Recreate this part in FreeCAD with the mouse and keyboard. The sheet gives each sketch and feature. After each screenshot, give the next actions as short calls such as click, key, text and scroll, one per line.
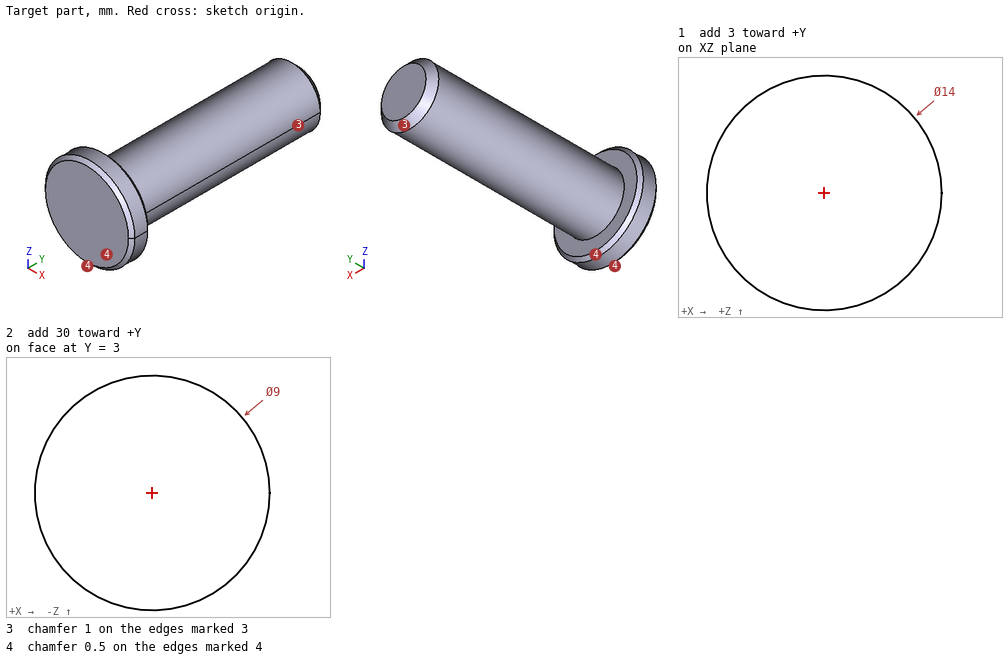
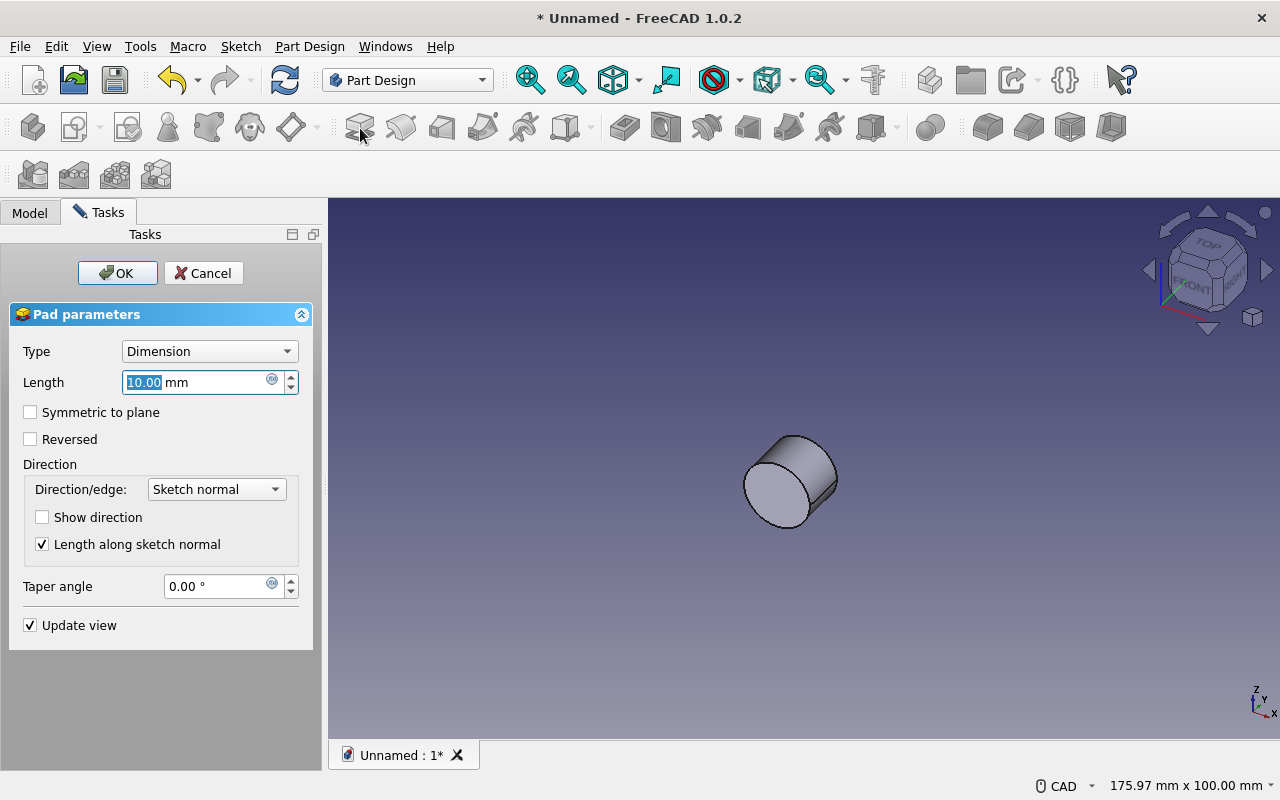
text(3)
key(Tab)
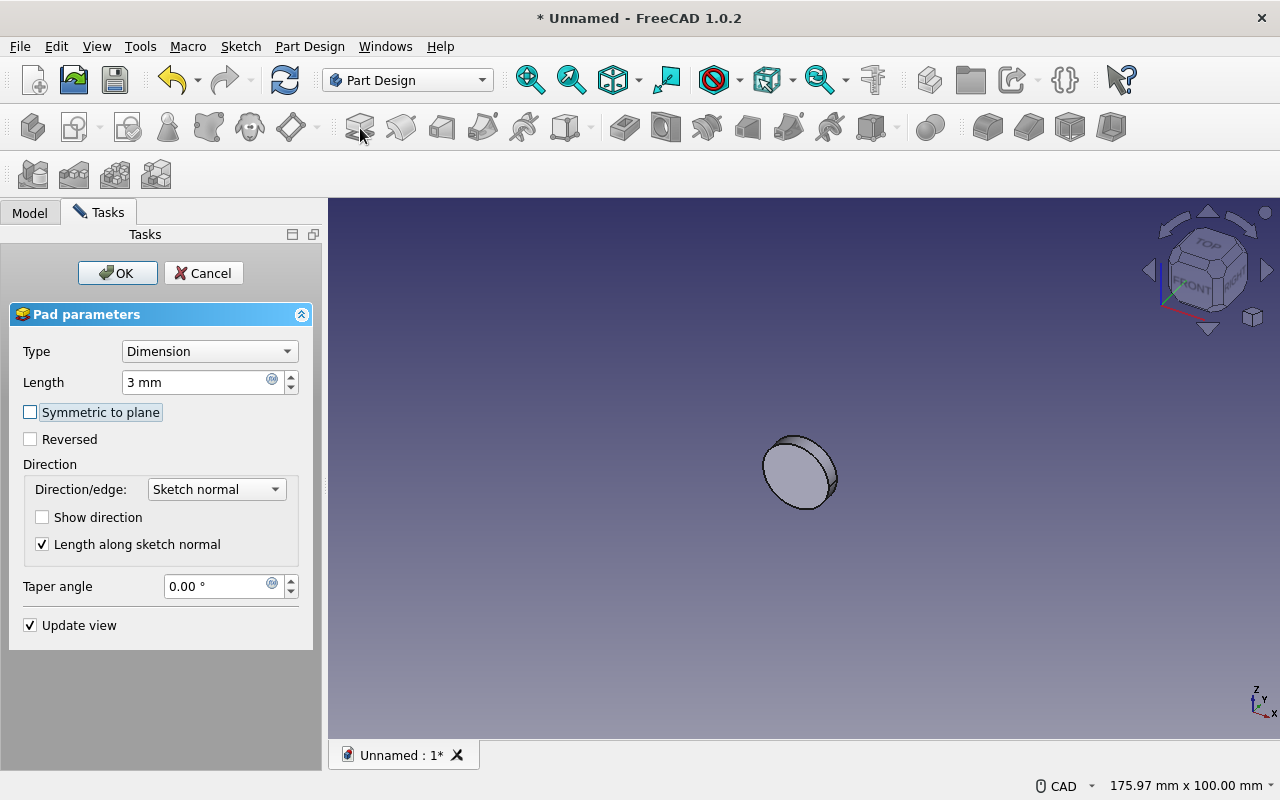
click(31, 439)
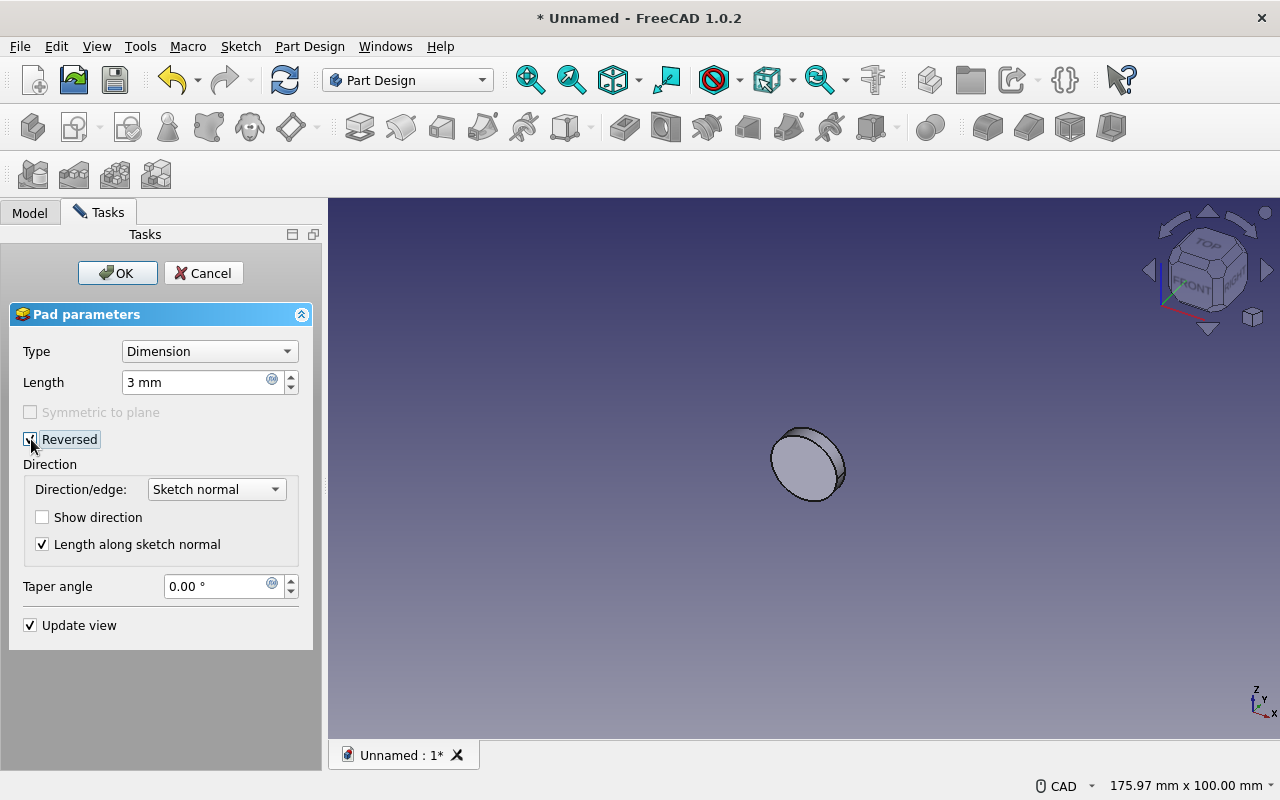
click(118, 273)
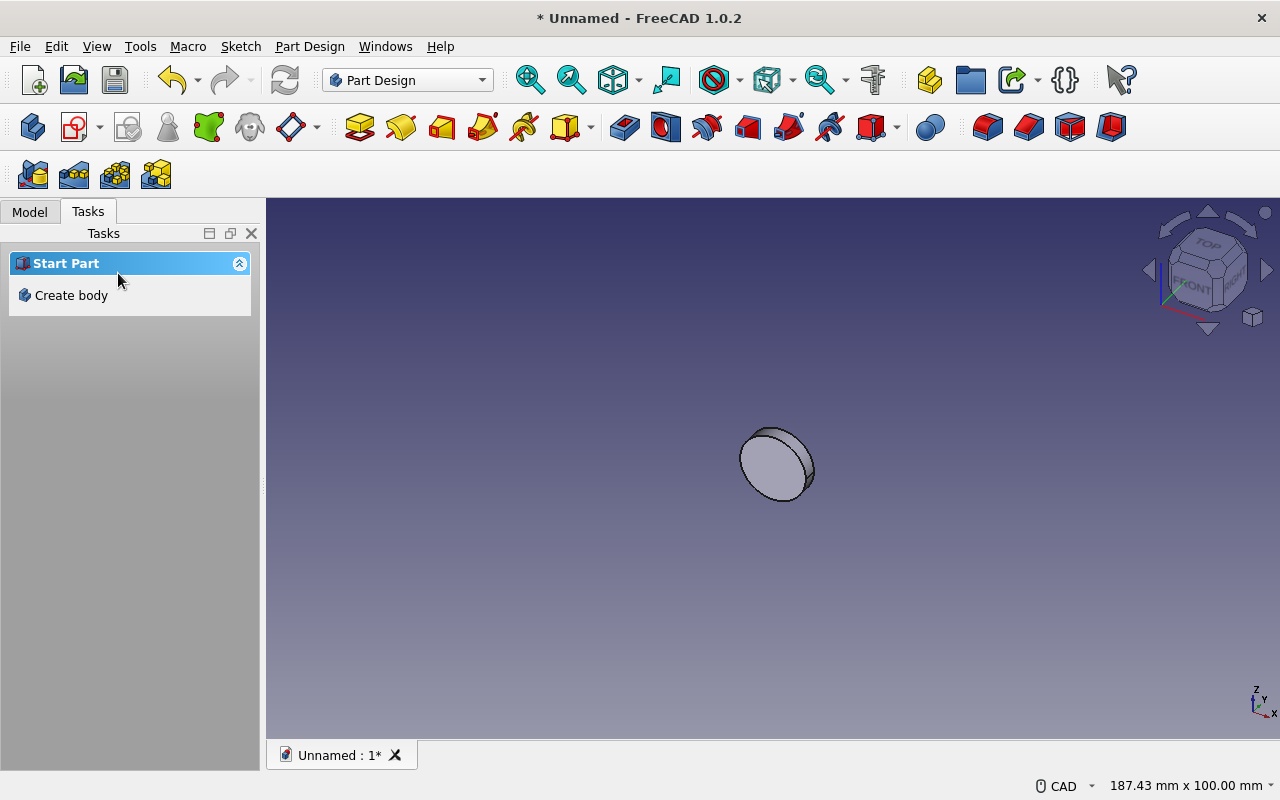
key(v)
key(f)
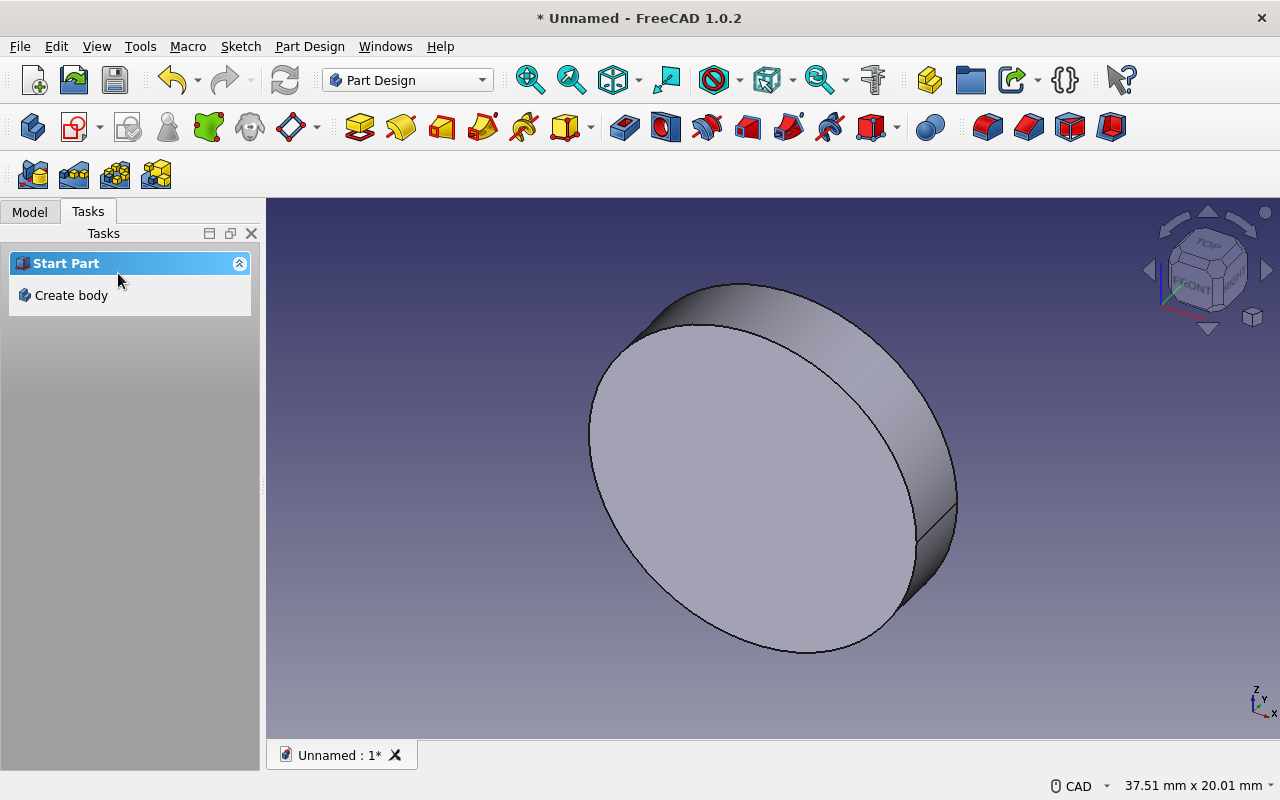
key(4)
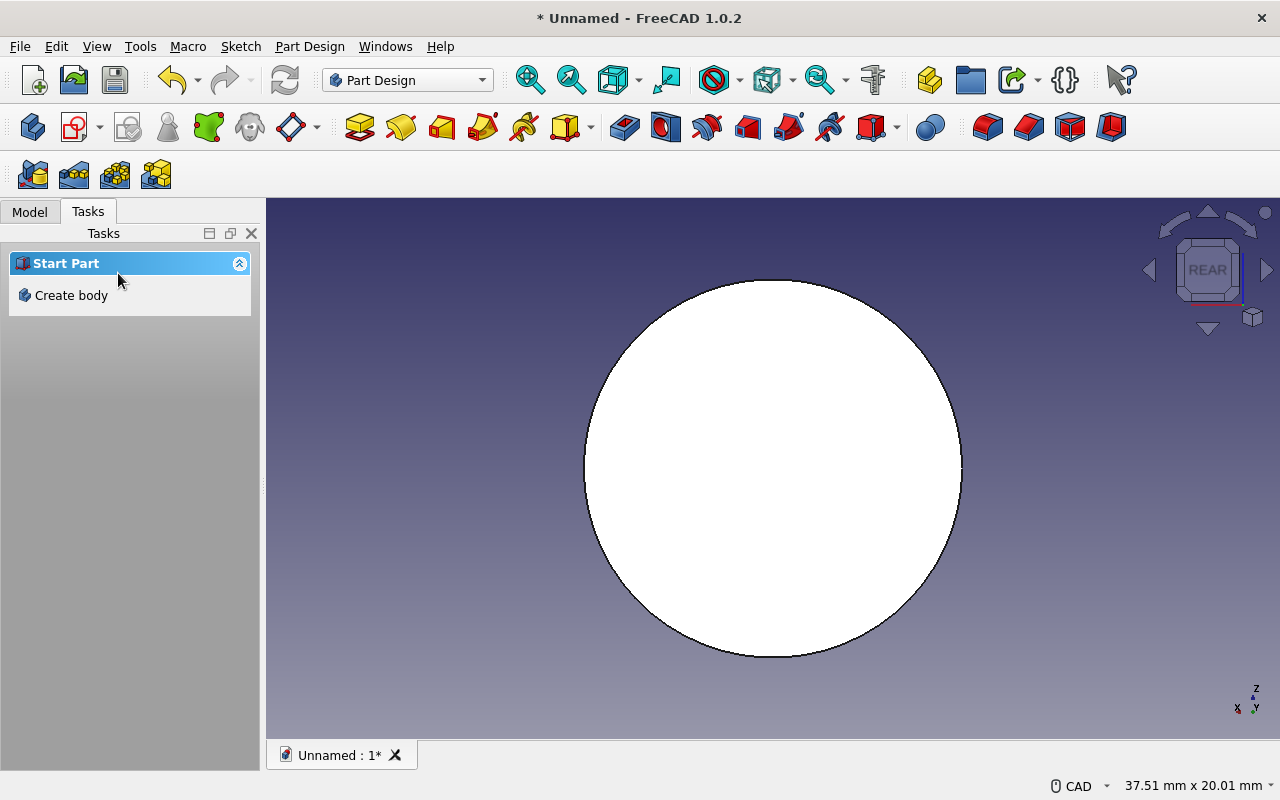
click(773, 468)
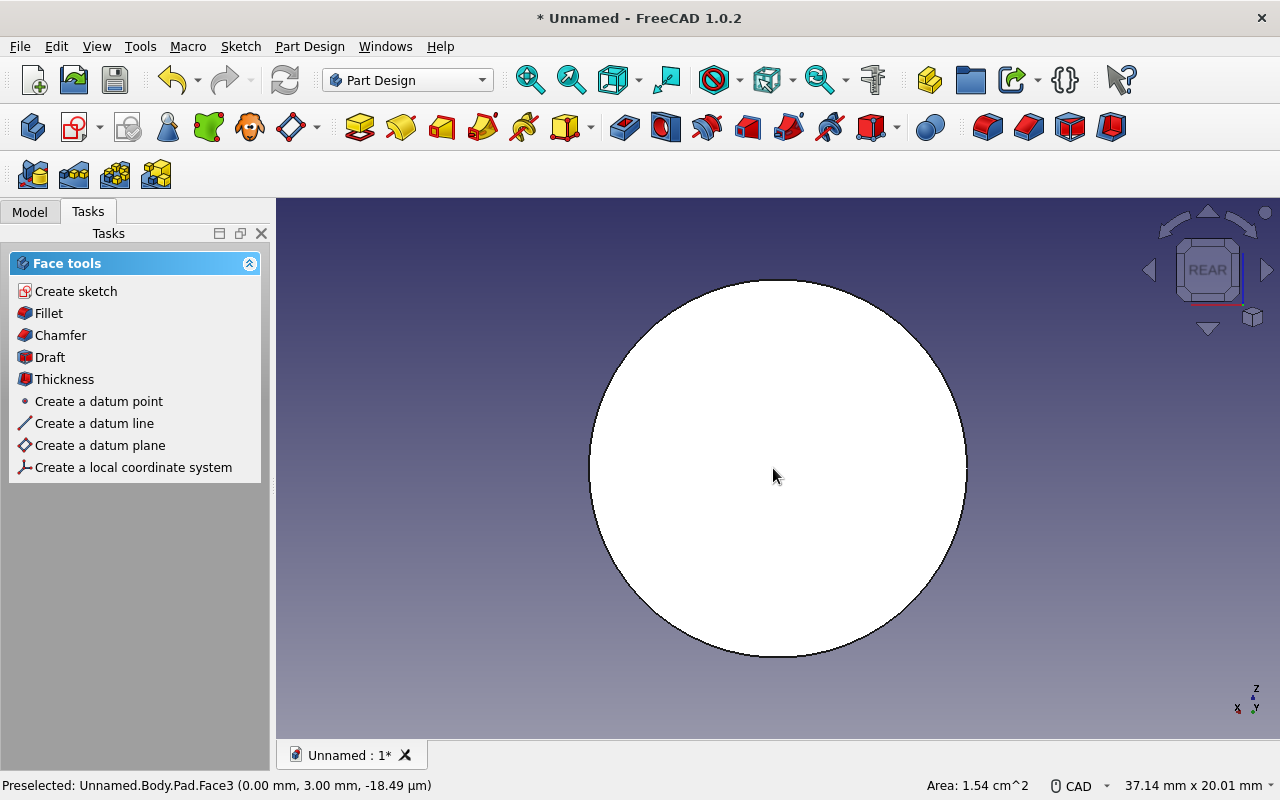
click(74, 128)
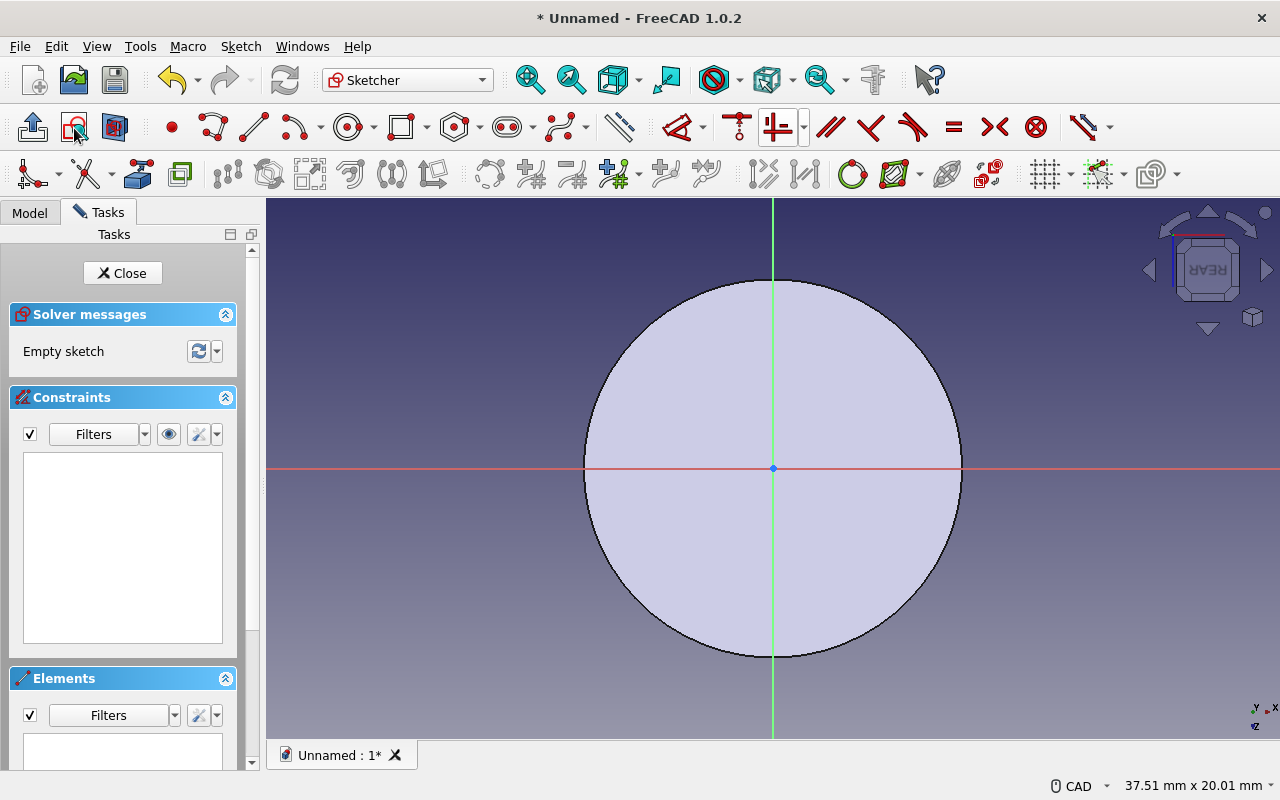
scroll(912, 469, up, 2)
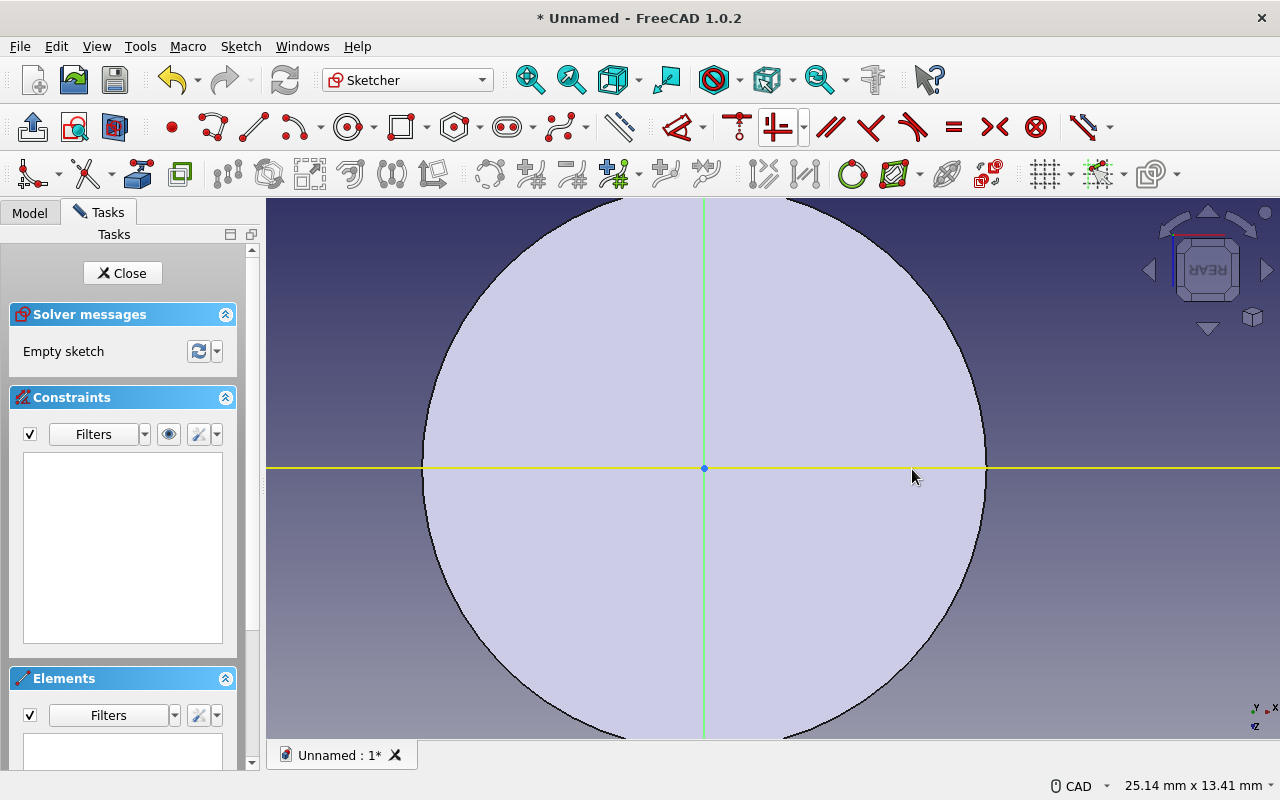
key(g)
key(c)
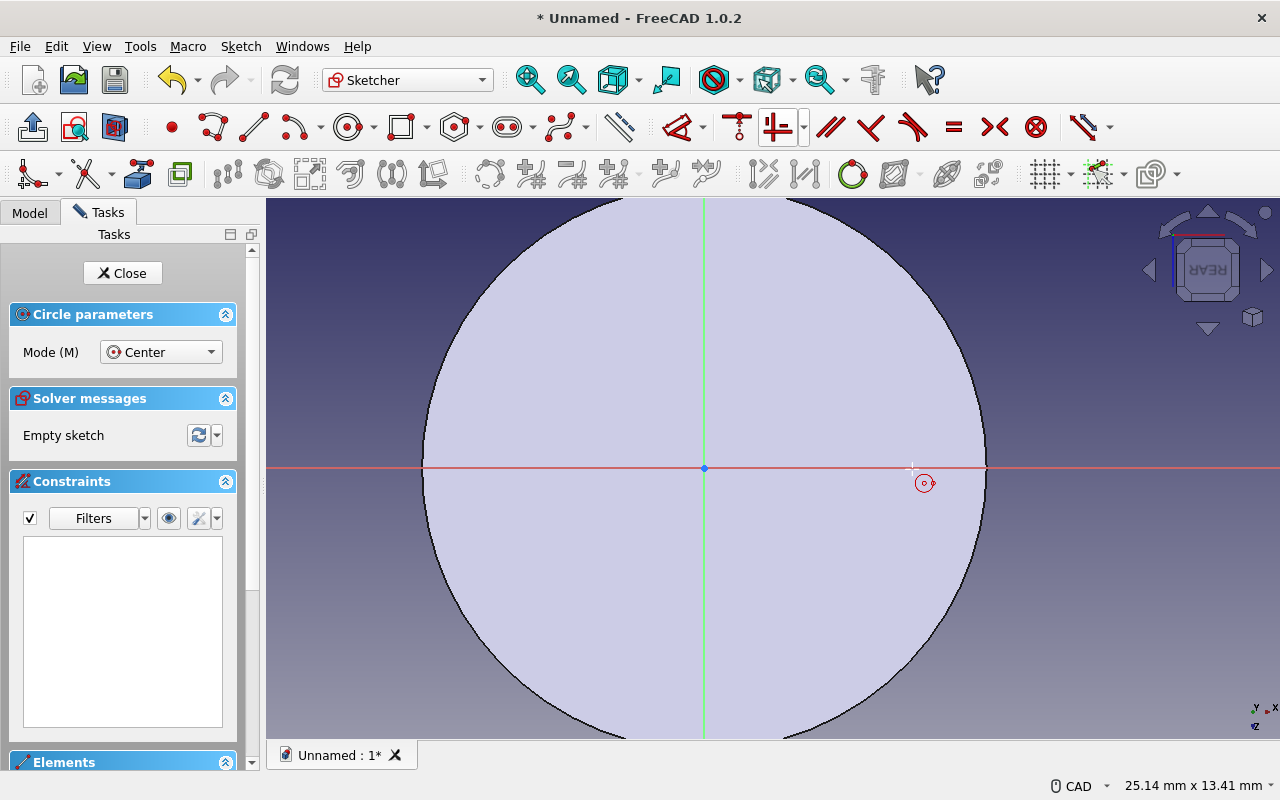
click(704, 468)
move(833, 340)